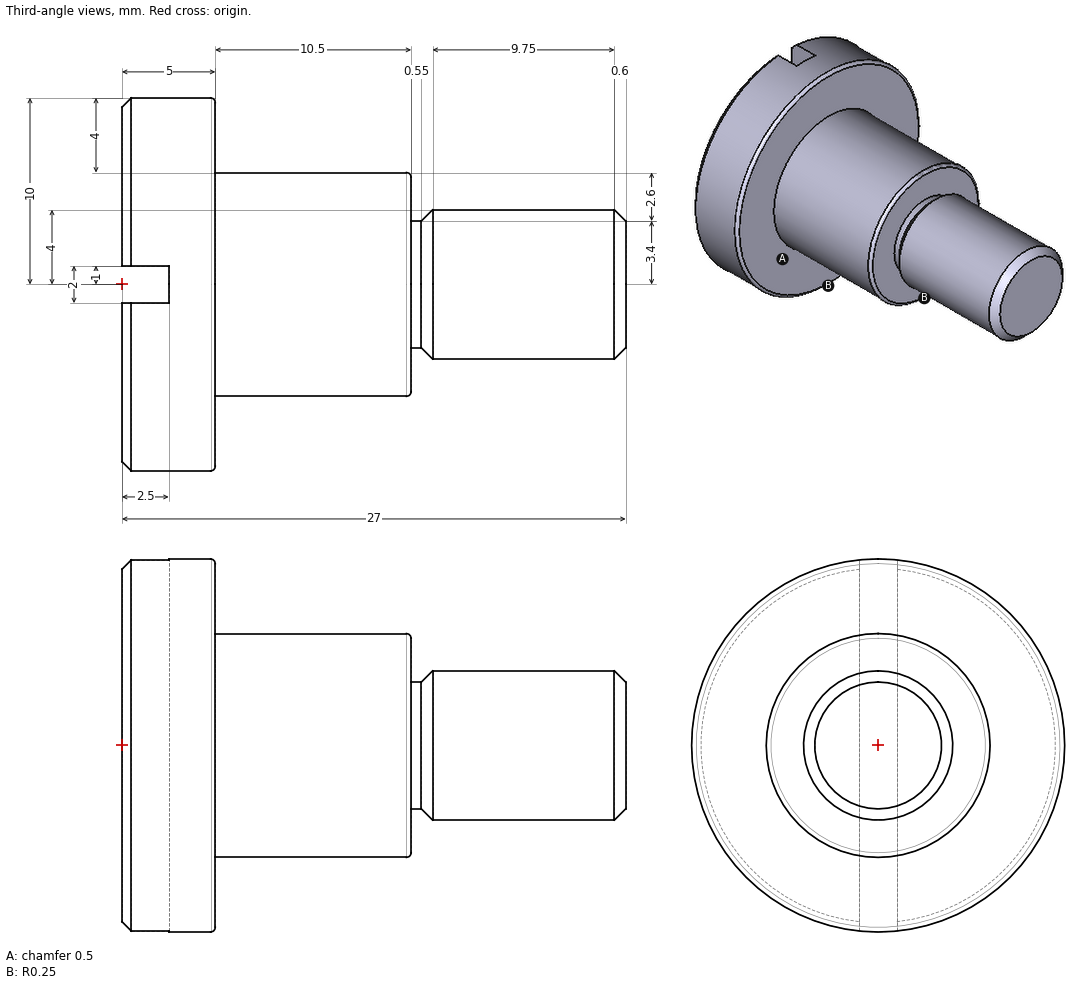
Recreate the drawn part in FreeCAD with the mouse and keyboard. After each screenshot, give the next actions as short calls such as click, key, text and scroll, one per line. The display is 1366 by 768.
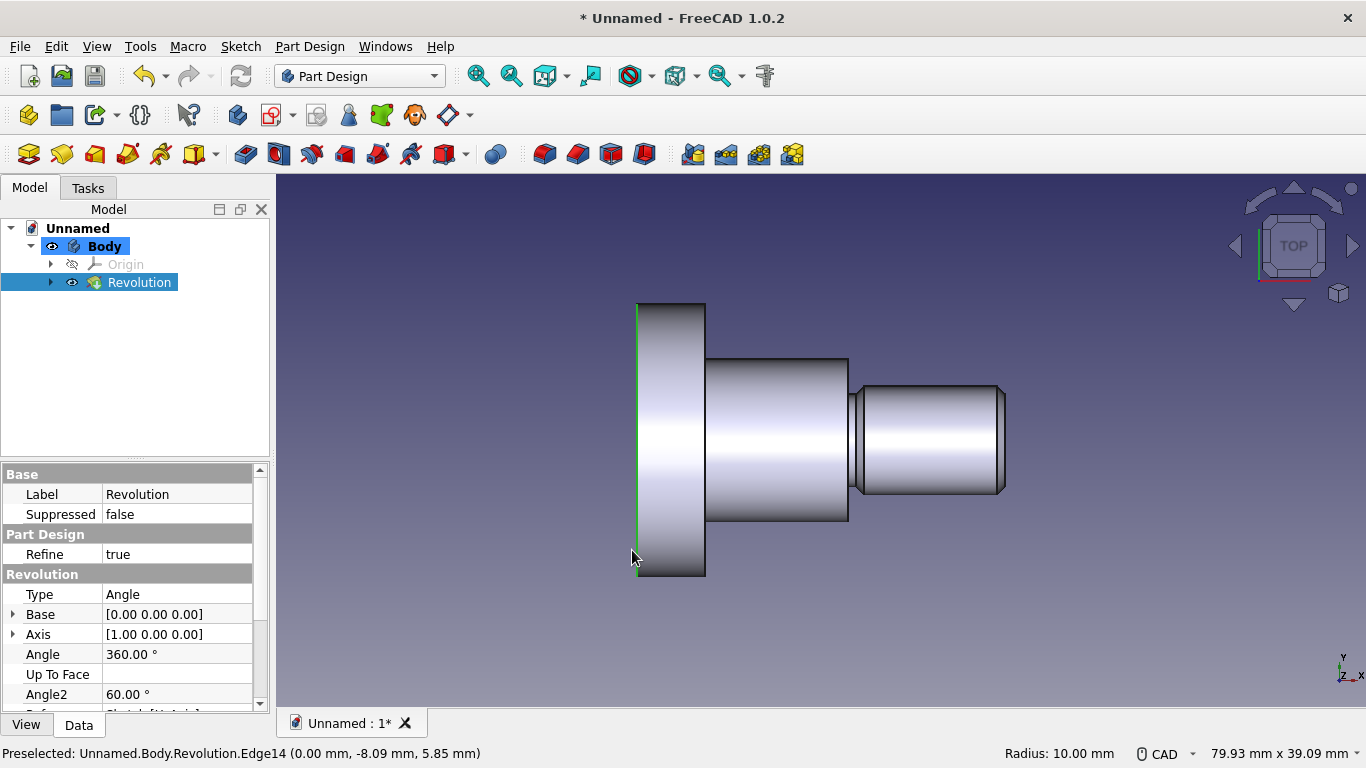
click(578, 154)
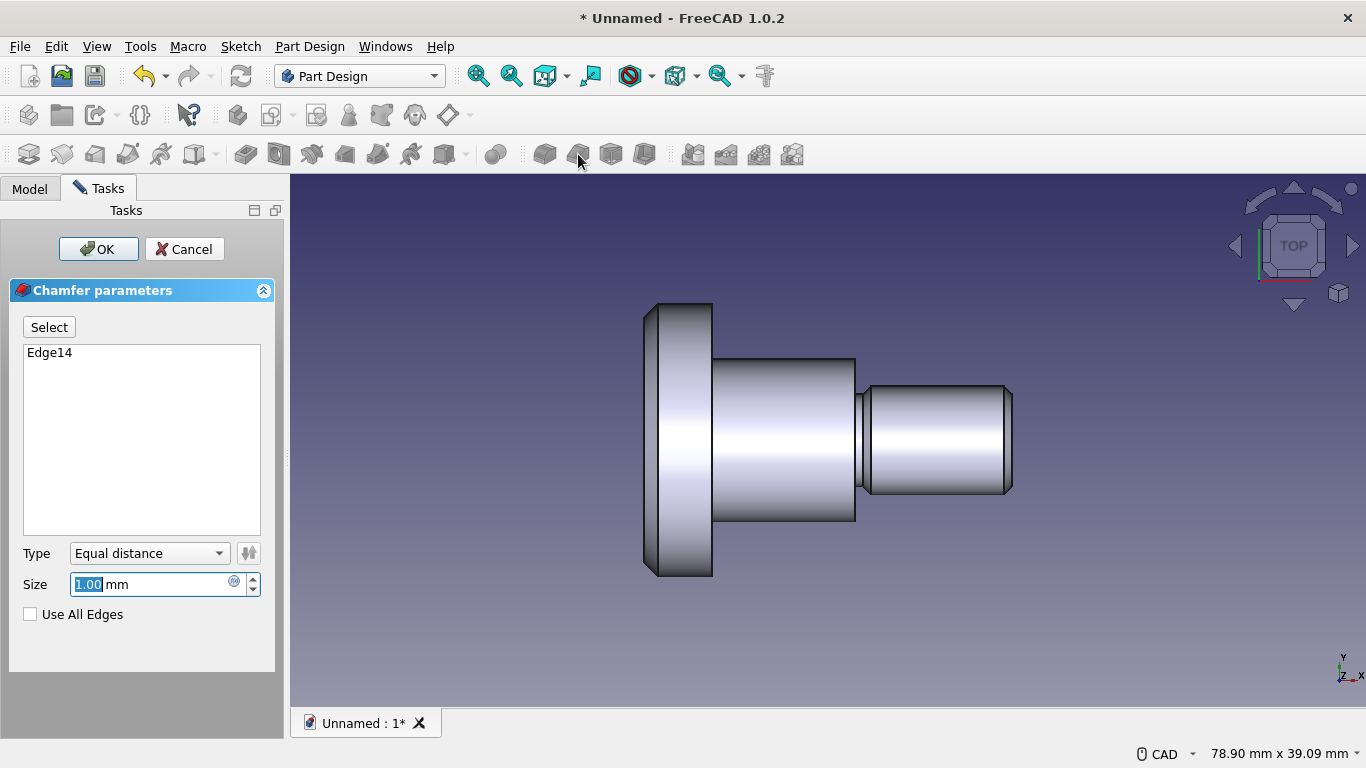
text(0.5)
key(Tab)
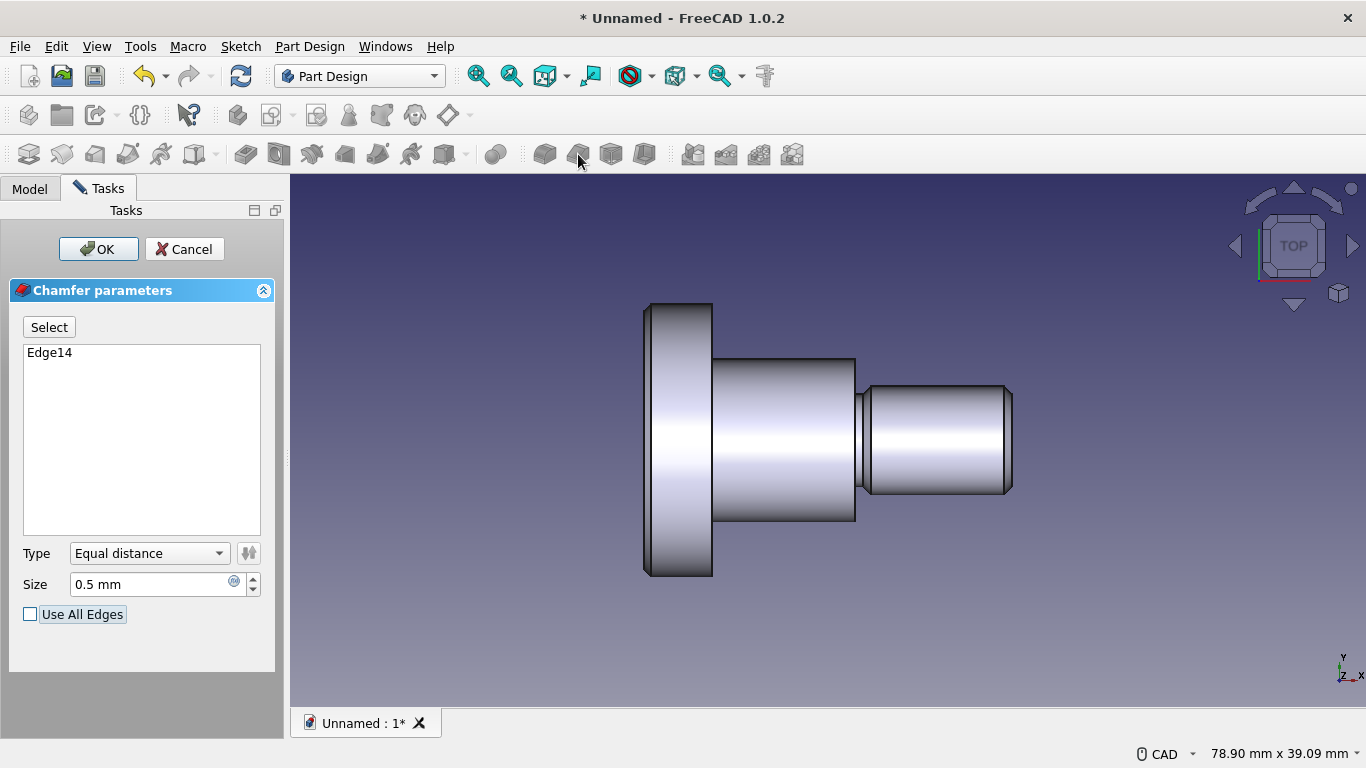
click(99, 249)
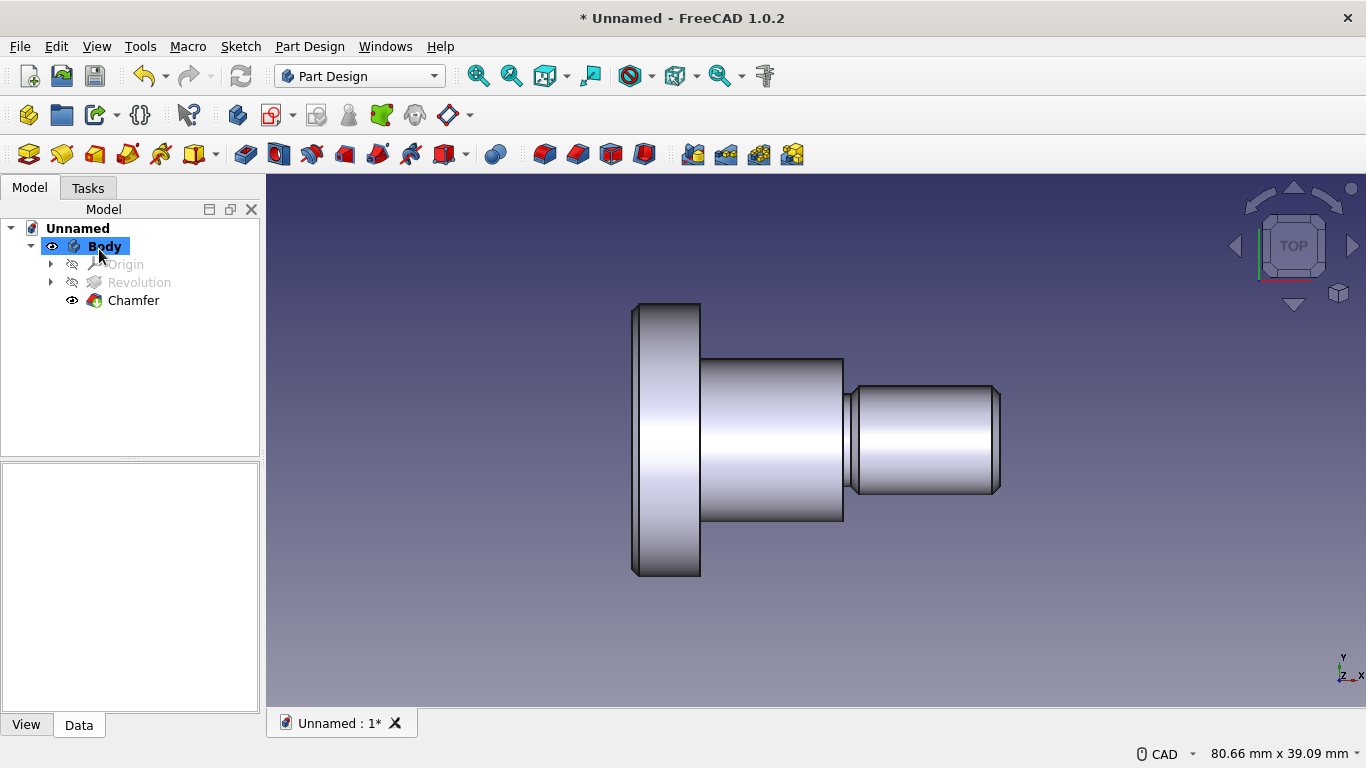
click(270, 116)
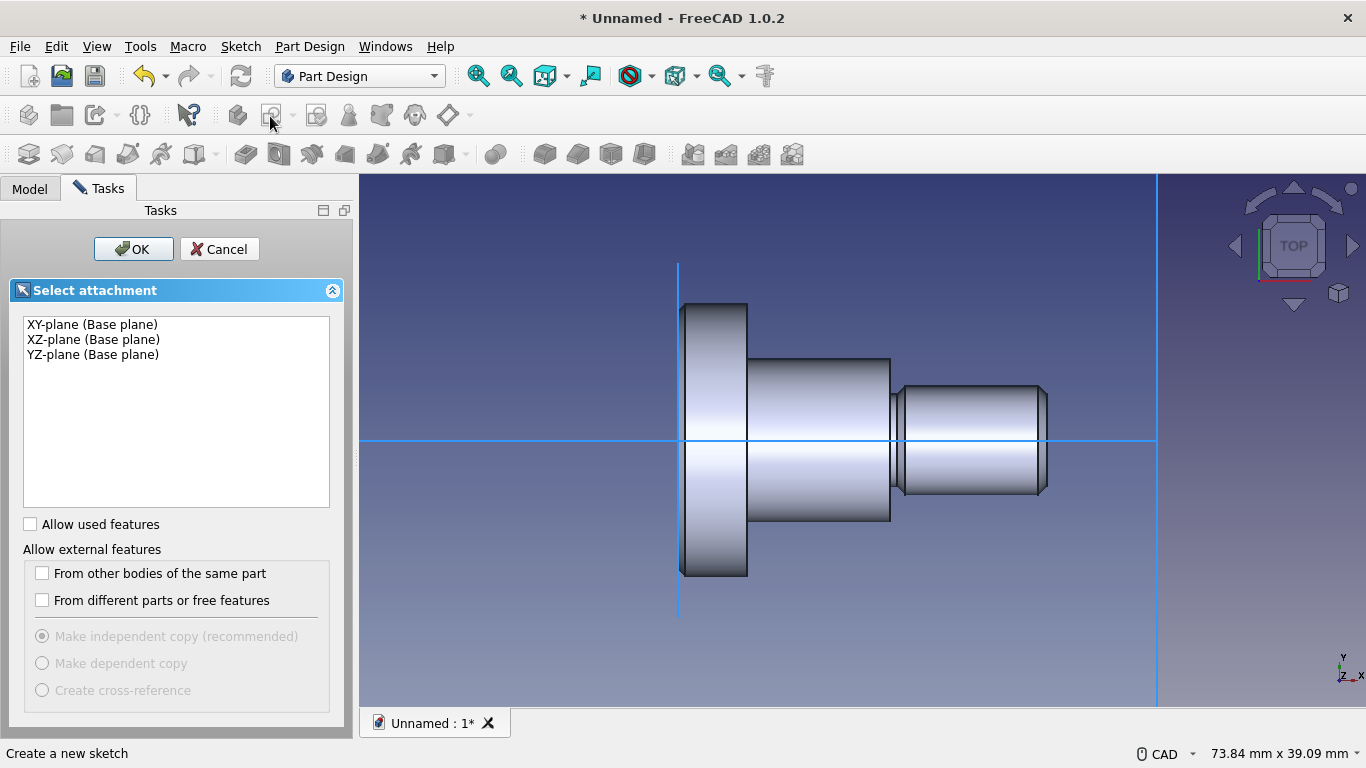
click(84, 324)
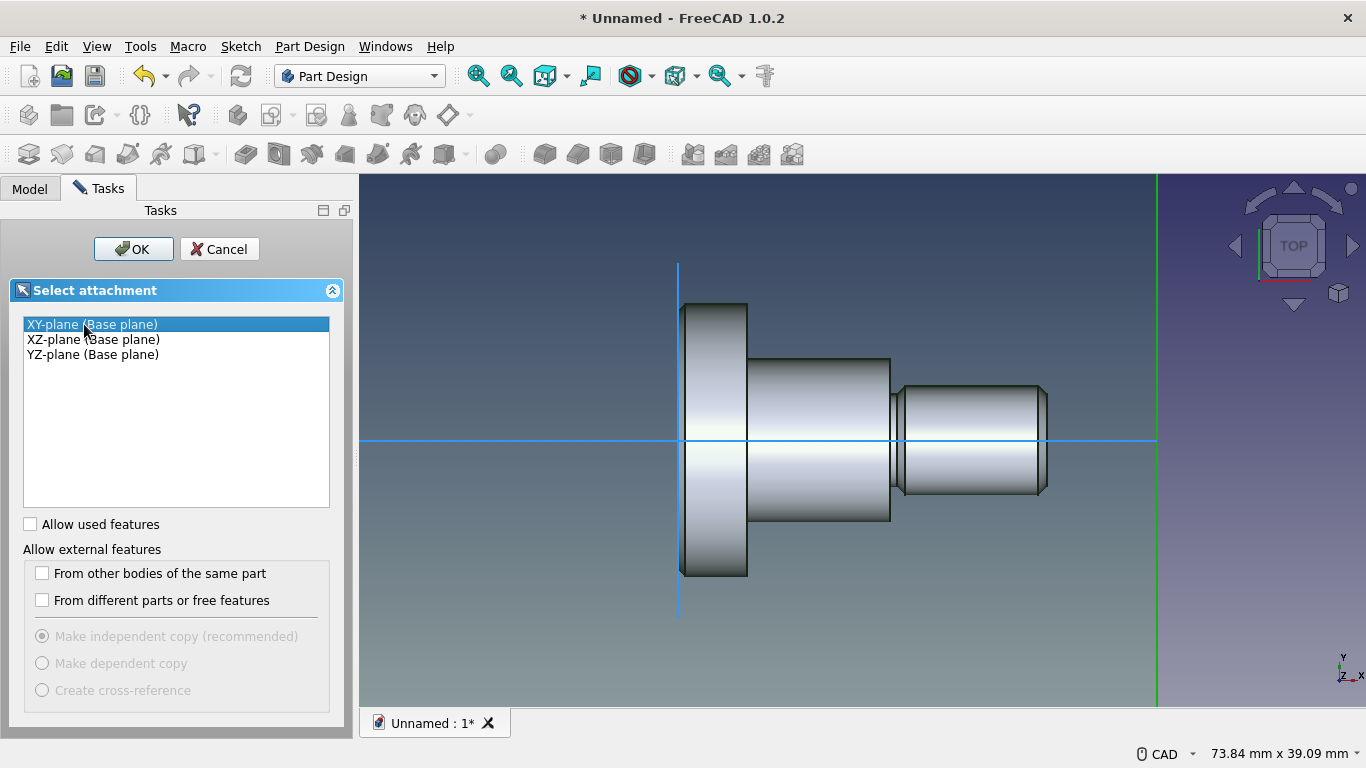
click(134, 249)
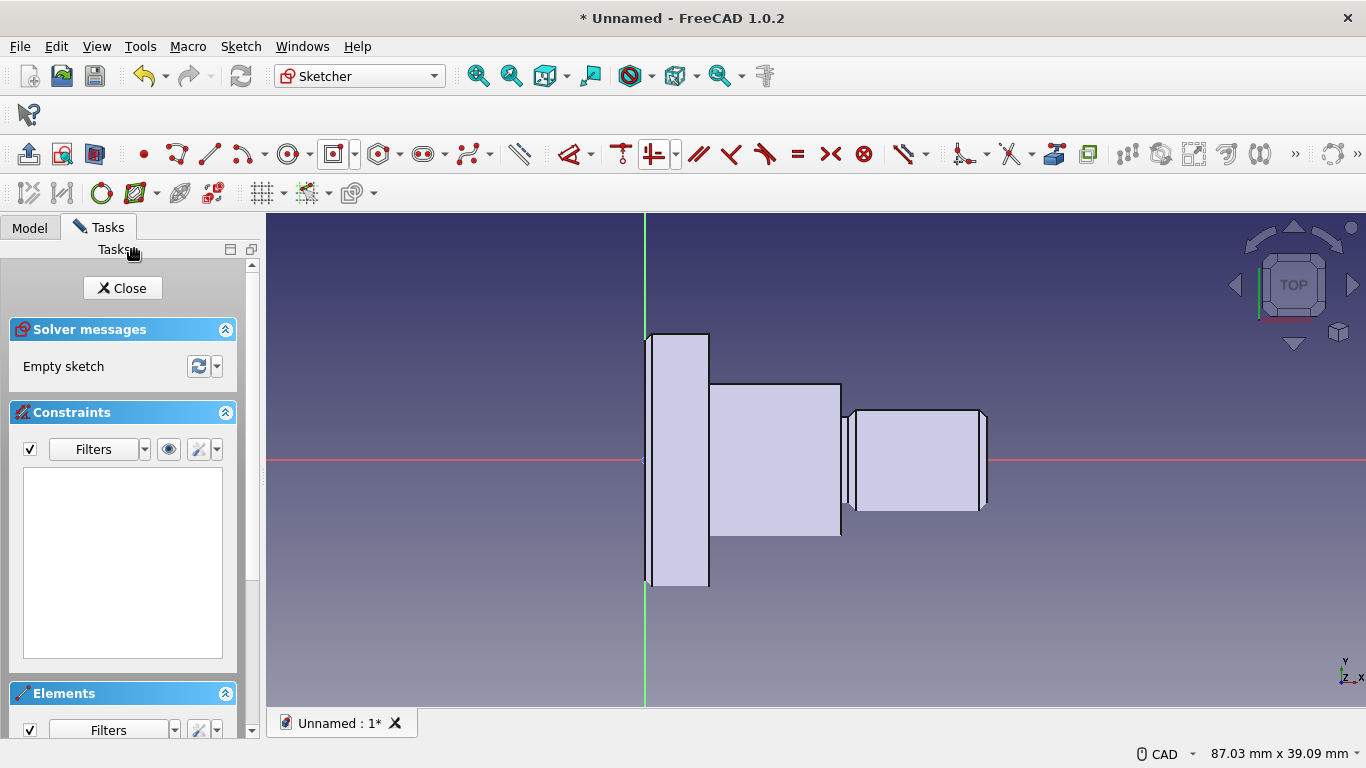
click(95, 154)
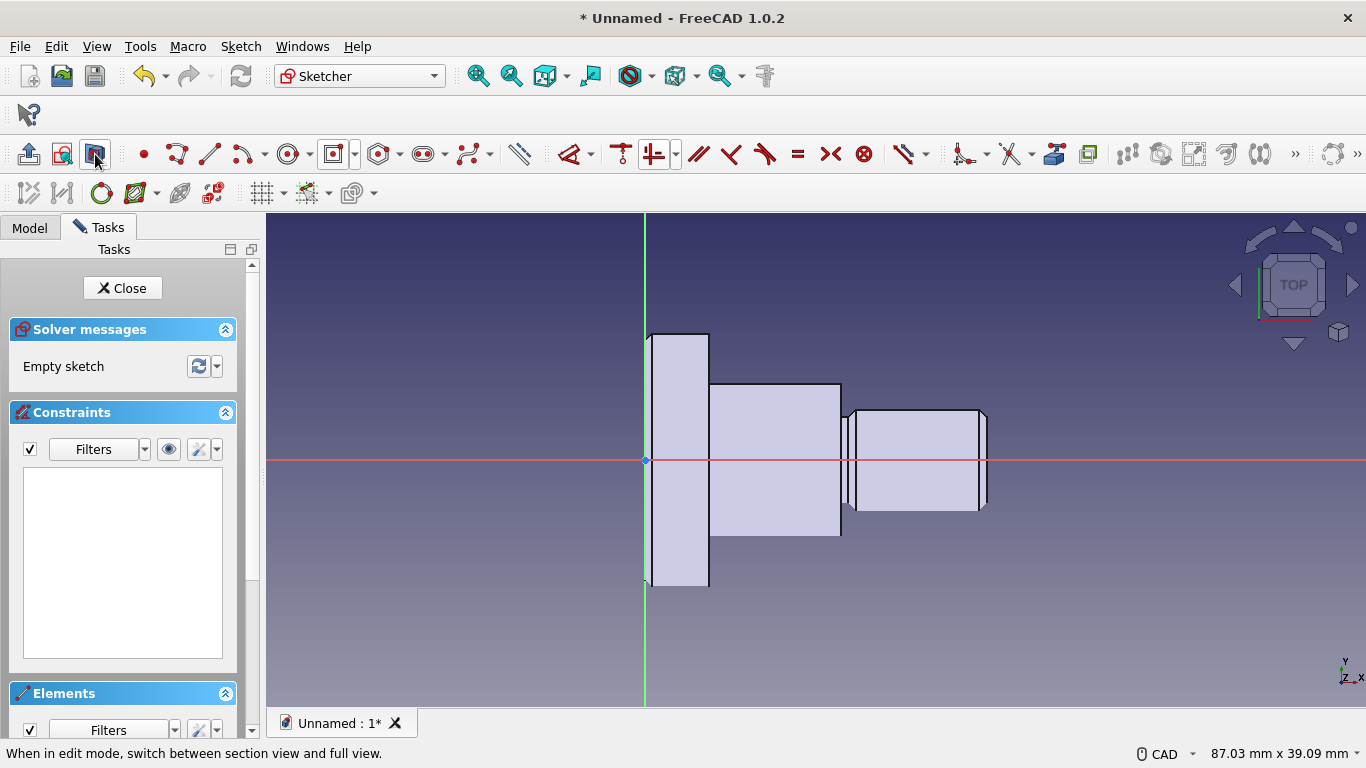
scroll(654, 460, up, 13)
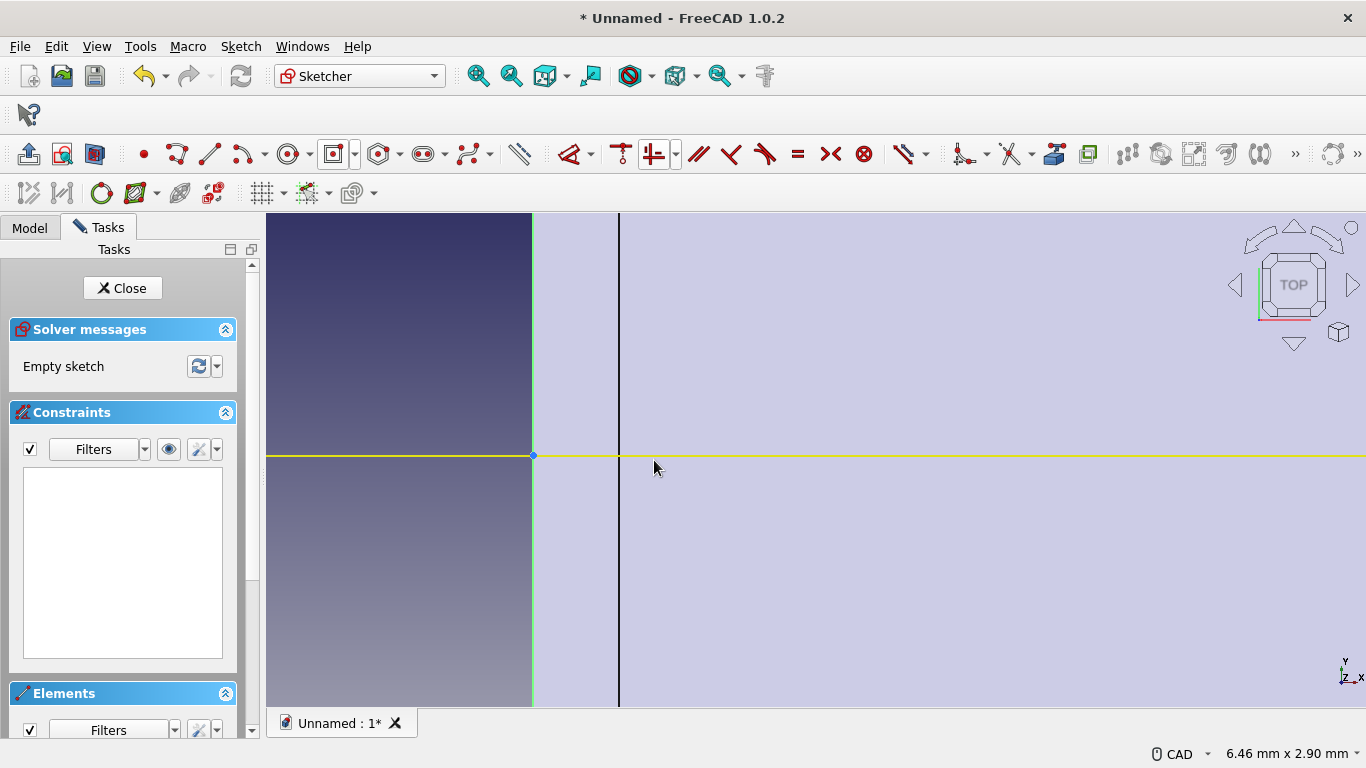
click(354, 154)